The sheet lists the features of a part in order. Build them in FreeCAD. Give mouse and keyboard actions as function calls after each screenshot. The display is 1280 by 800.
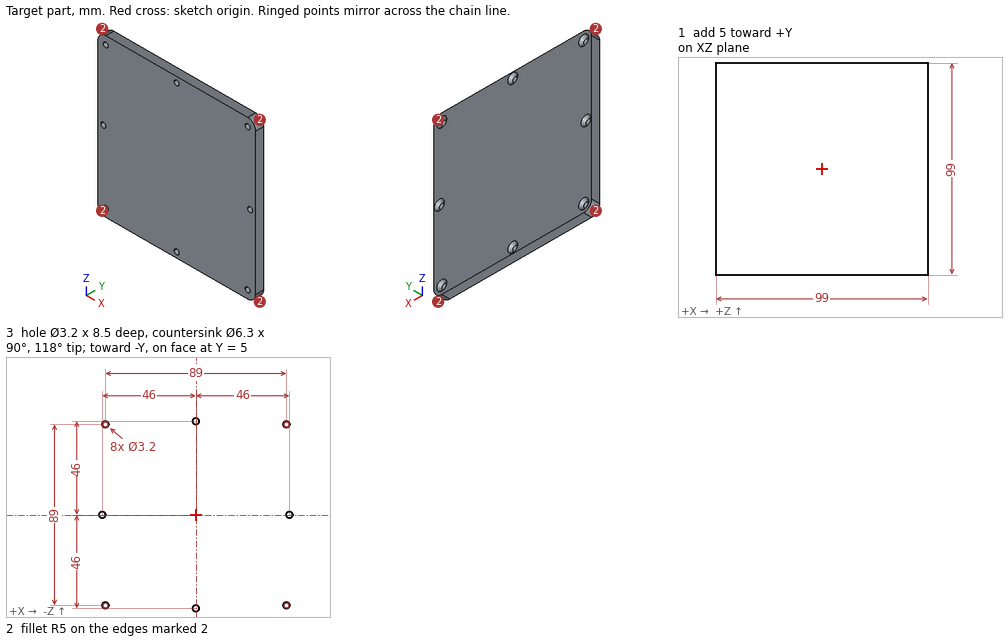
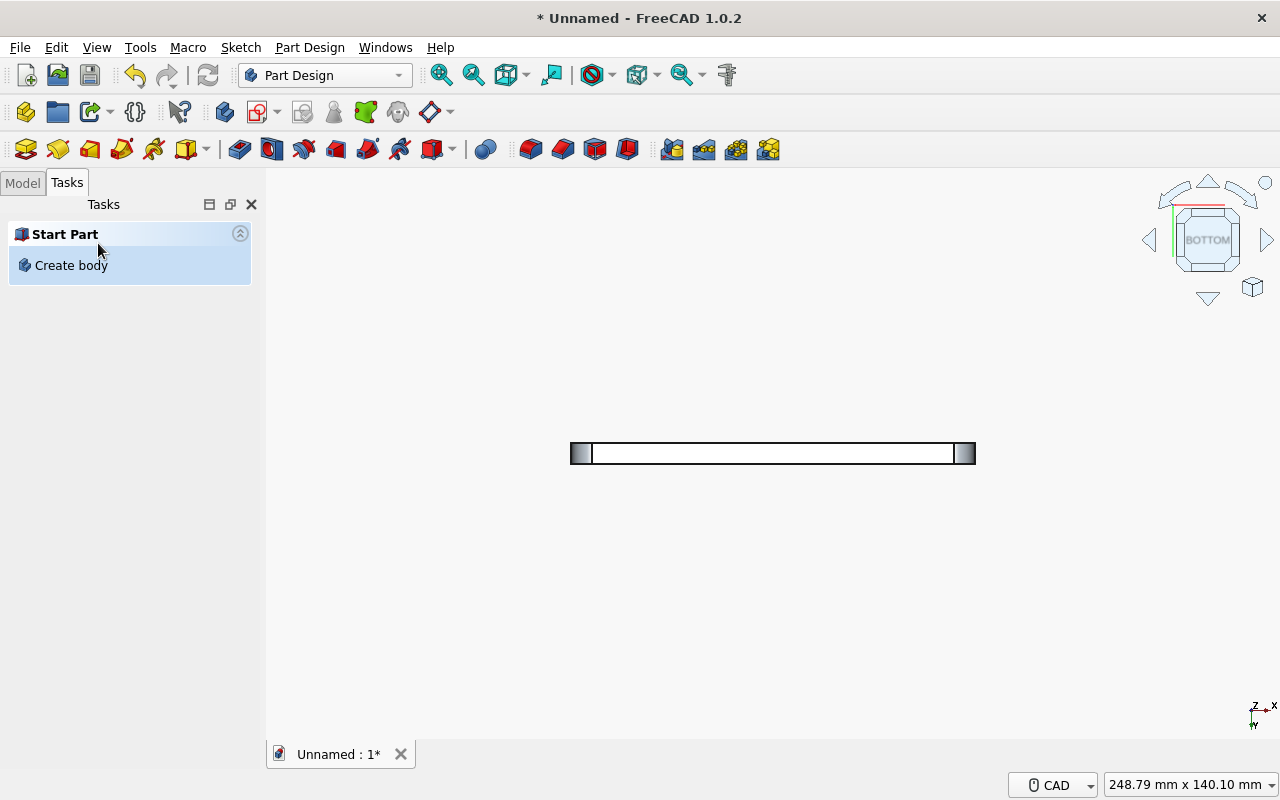
key(4)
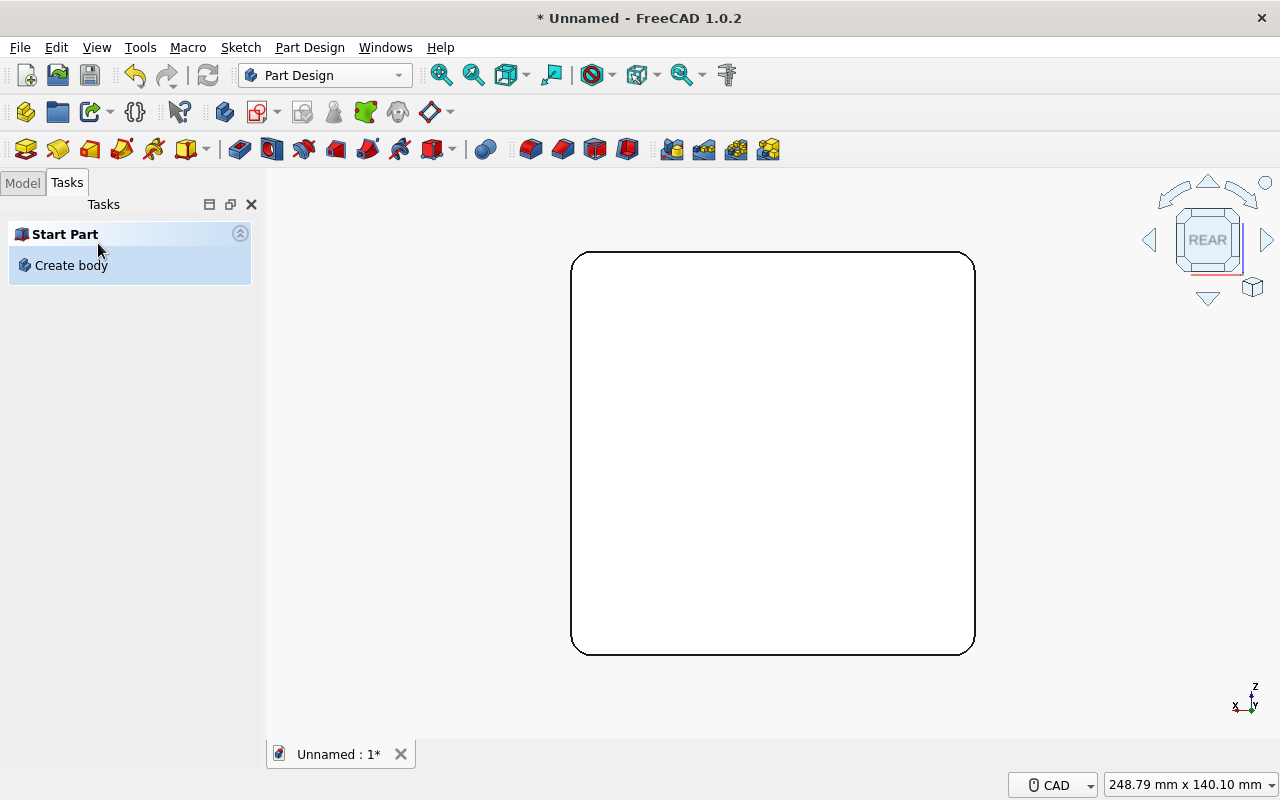
click(773, 452)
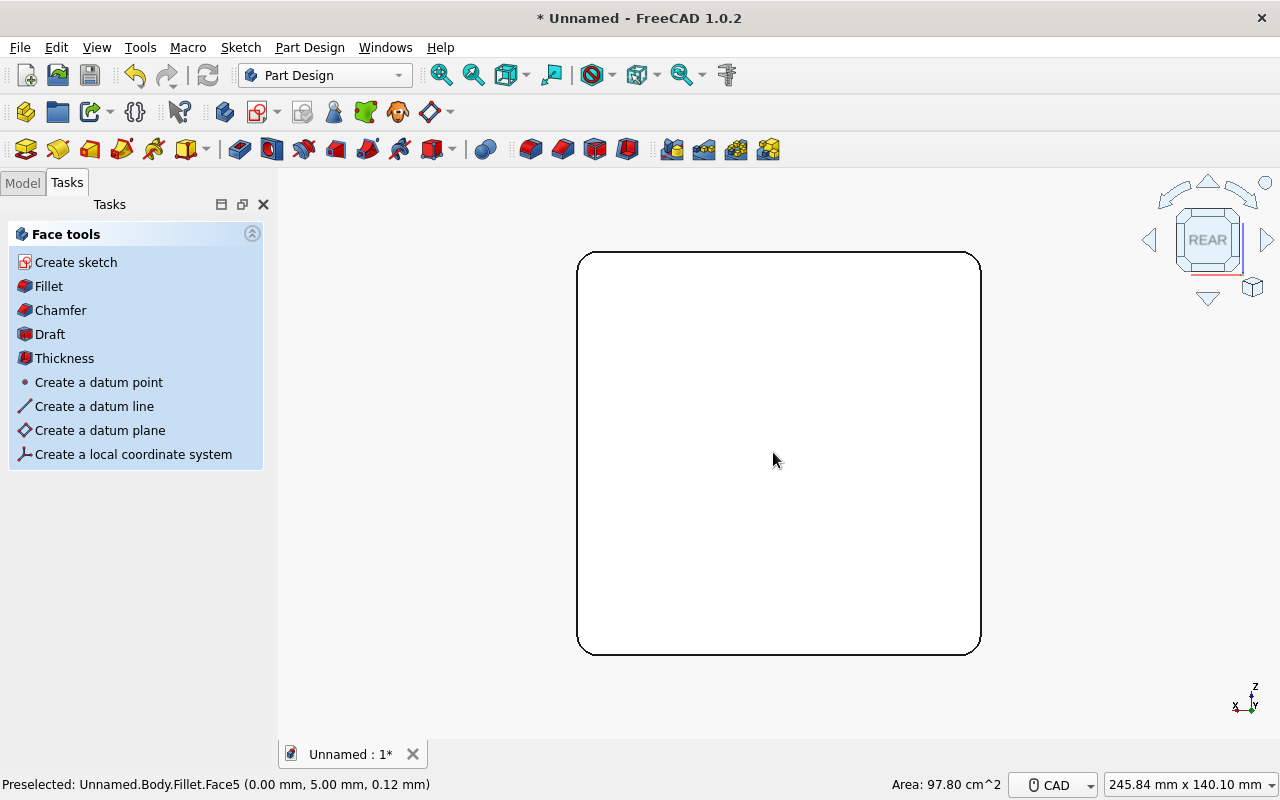
click(258, 112)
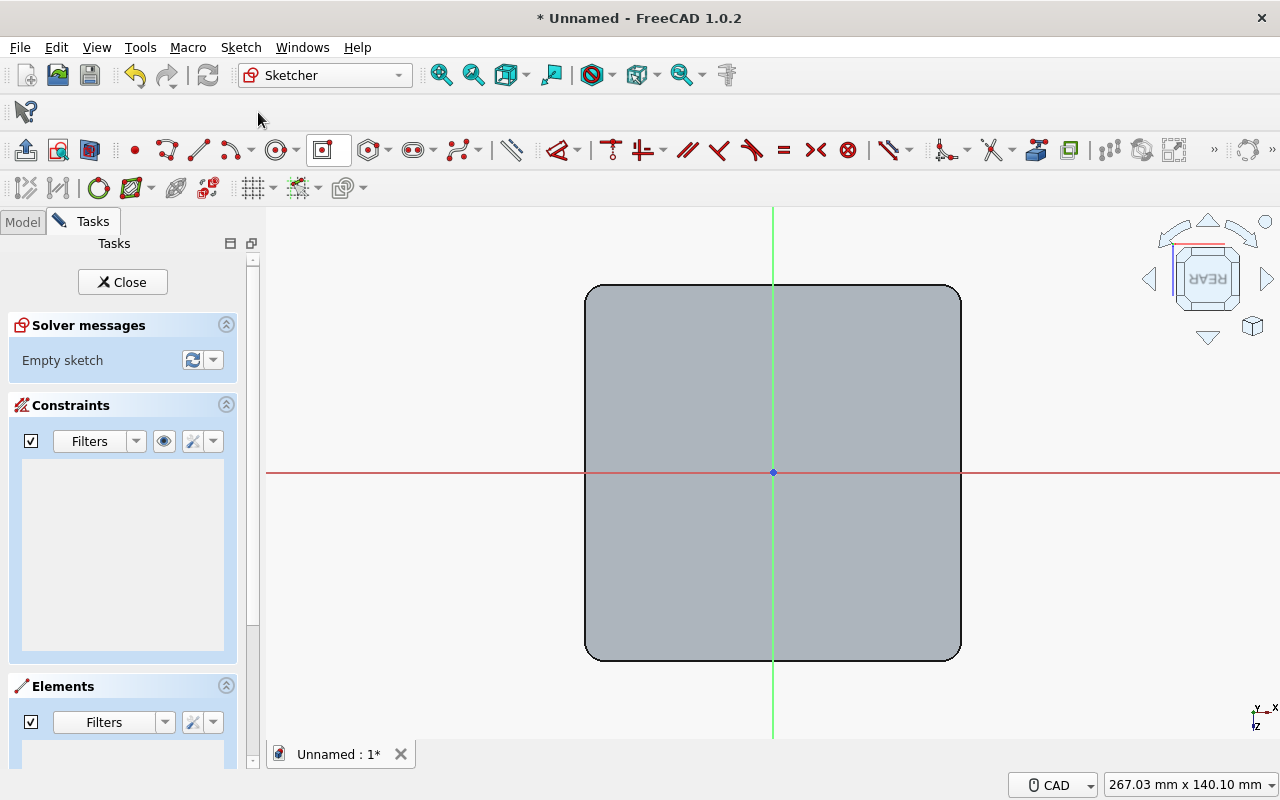
click(276, 150)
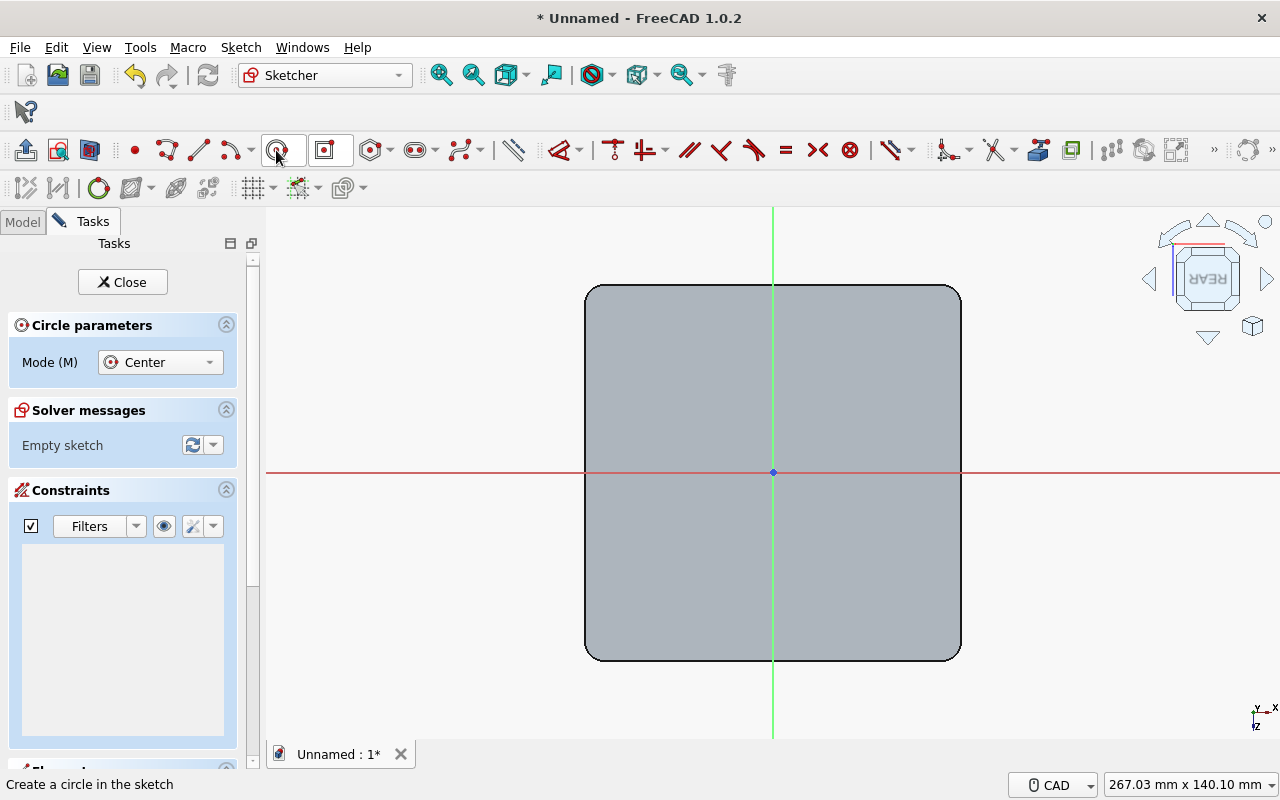
scroll(604, 304, up, 7)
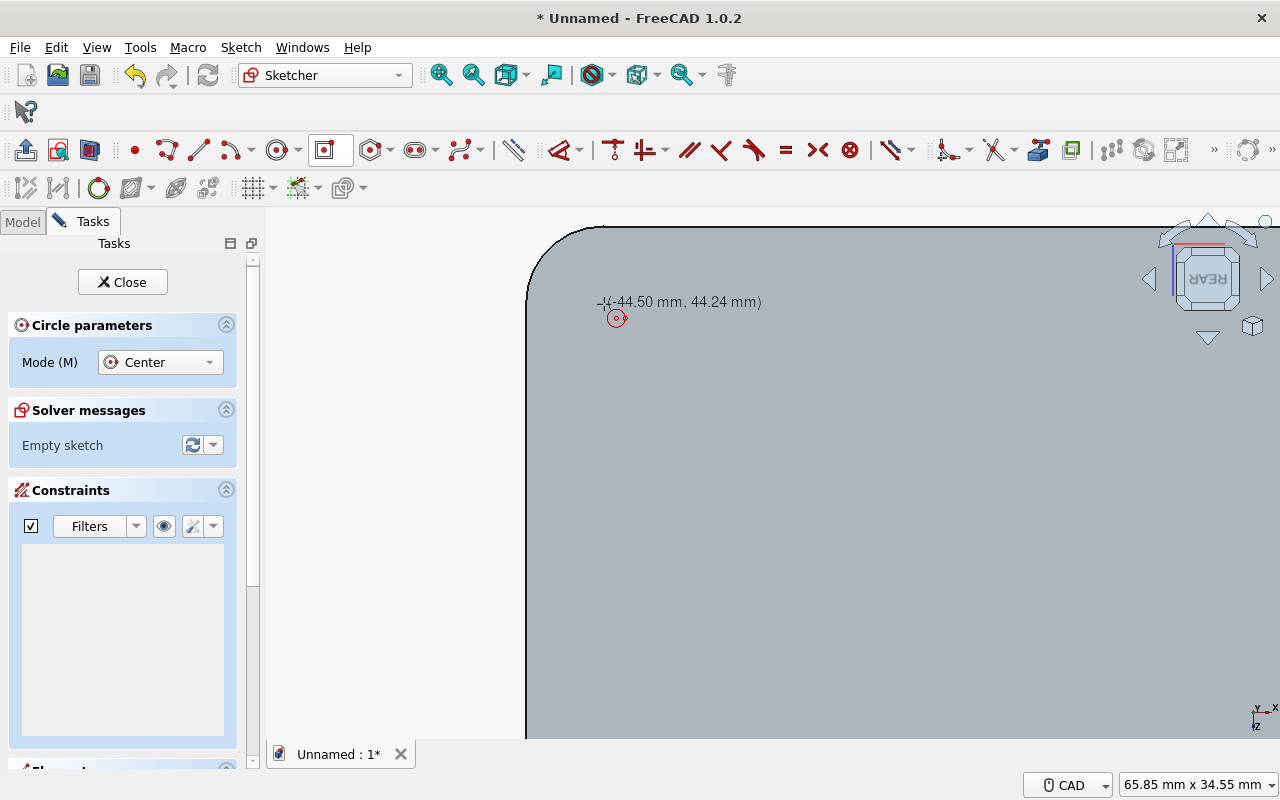
scroll(513, 304, down, 7)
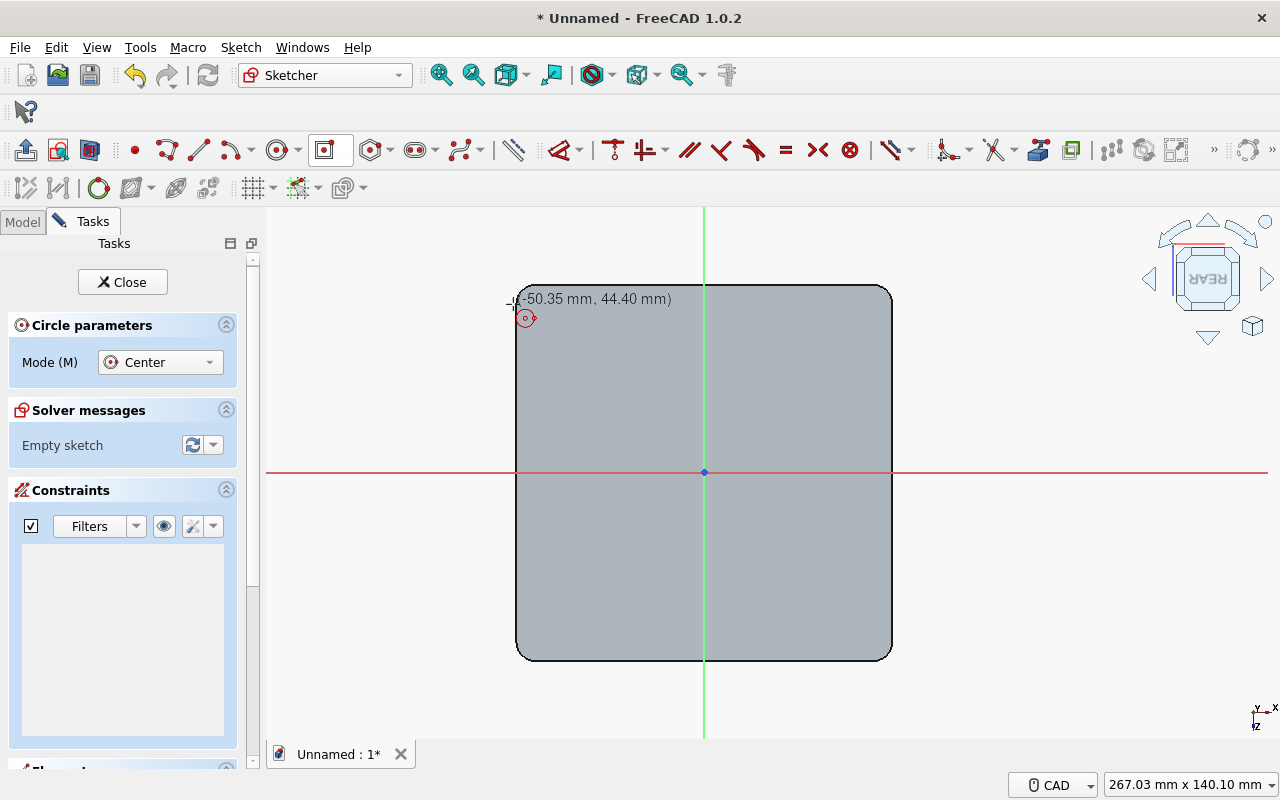
click(535, 304)
move(540, 300)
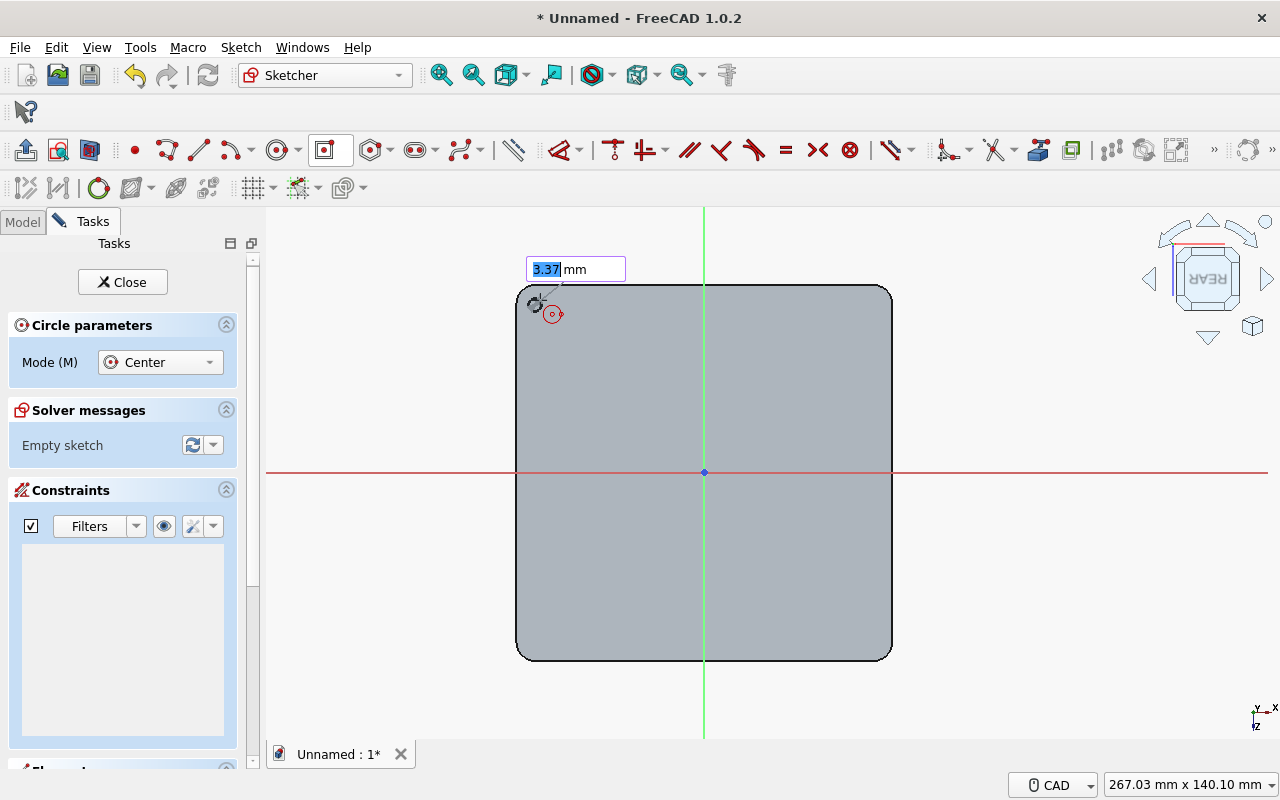
text(3.2)
key(Return)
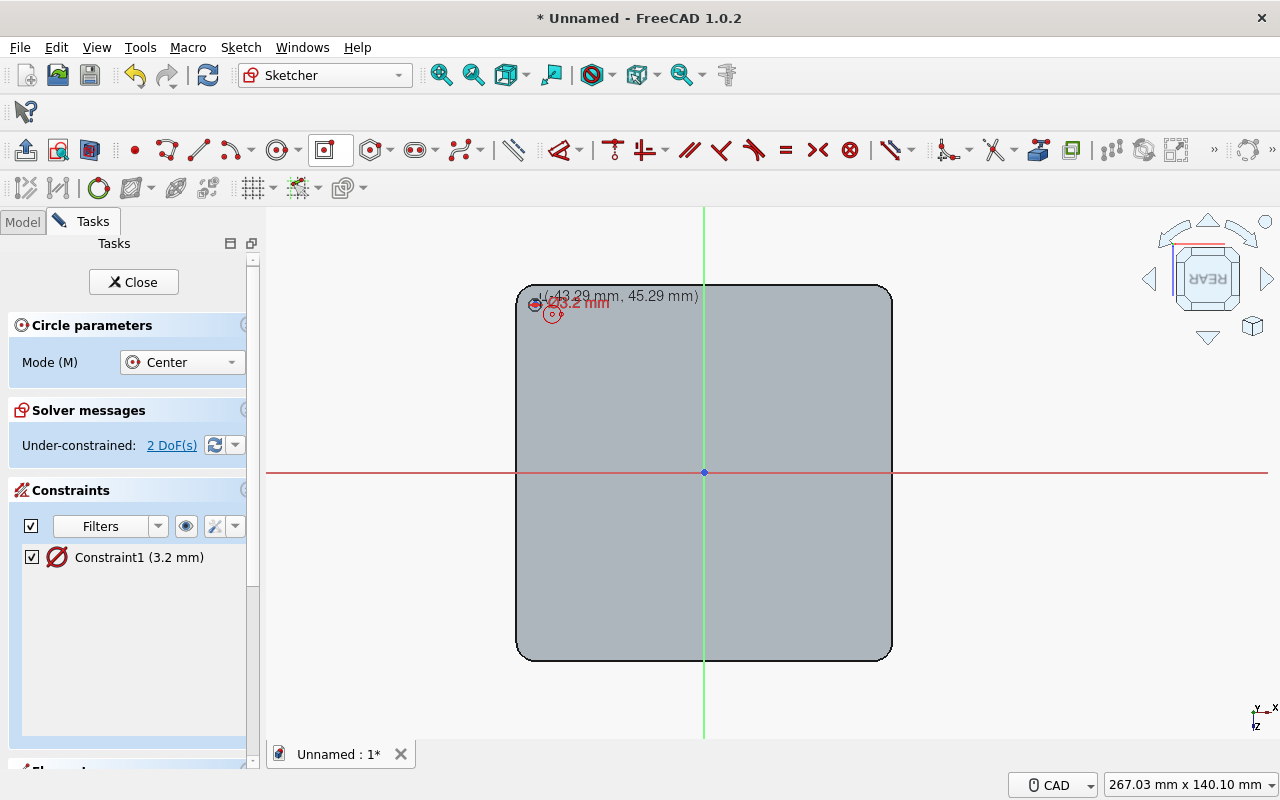
scroll(873, 304, up, 7)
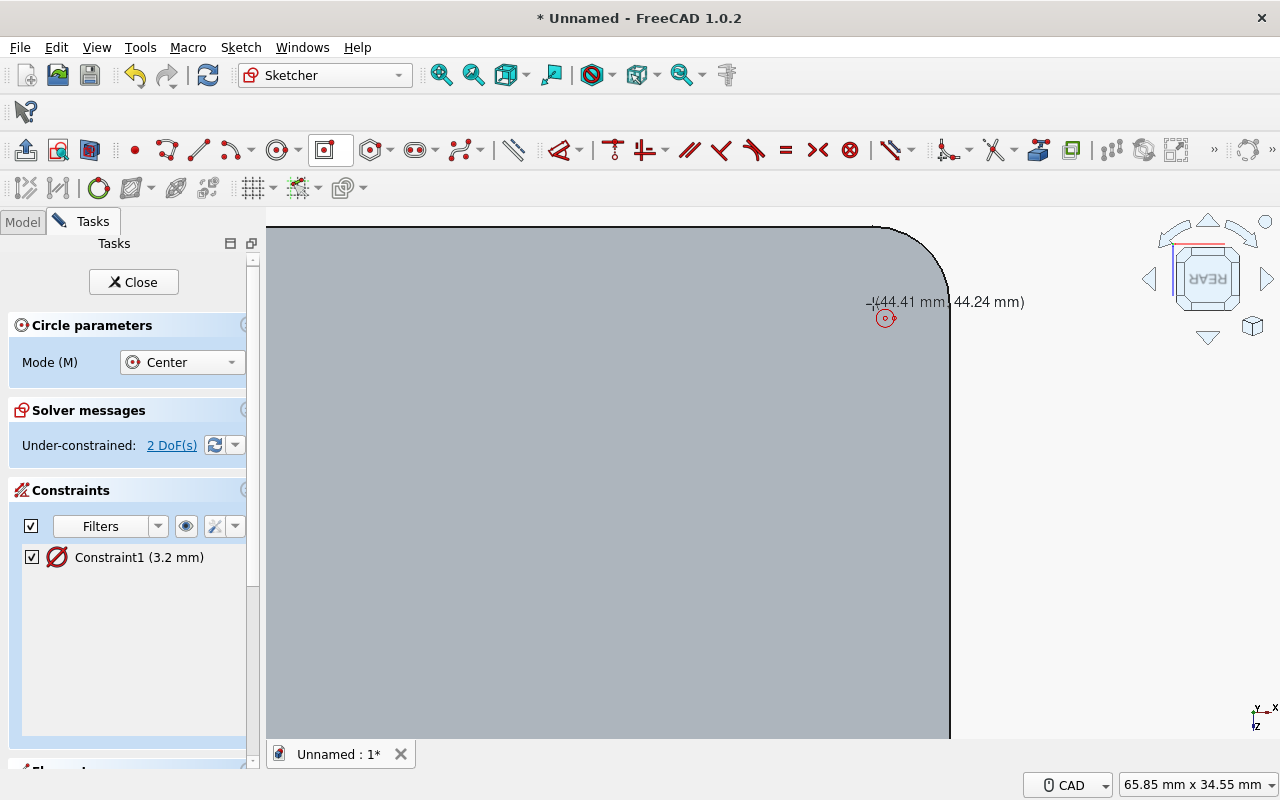
scroll(874, 304, down, 7)